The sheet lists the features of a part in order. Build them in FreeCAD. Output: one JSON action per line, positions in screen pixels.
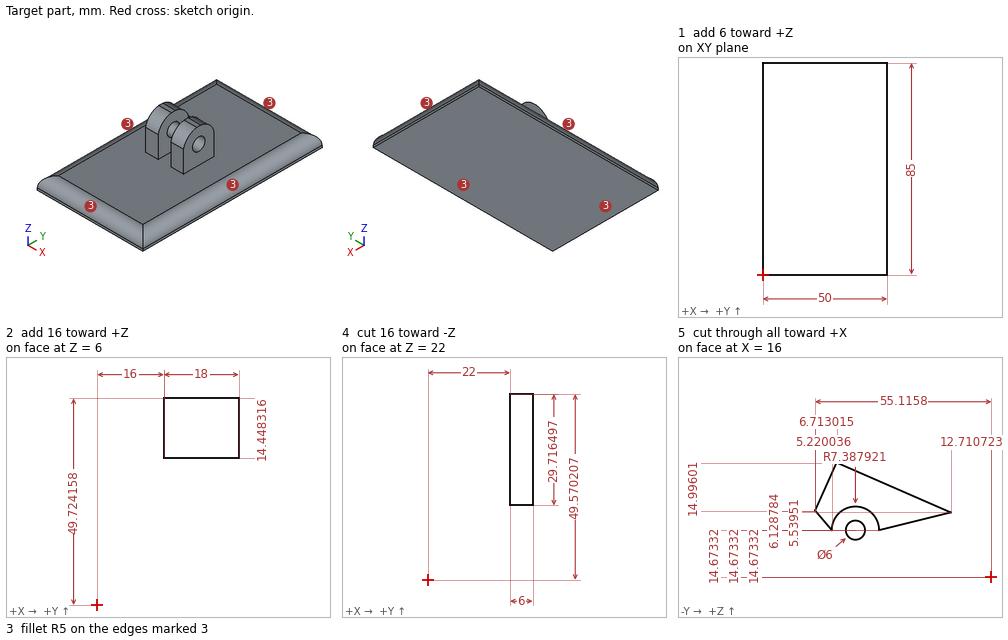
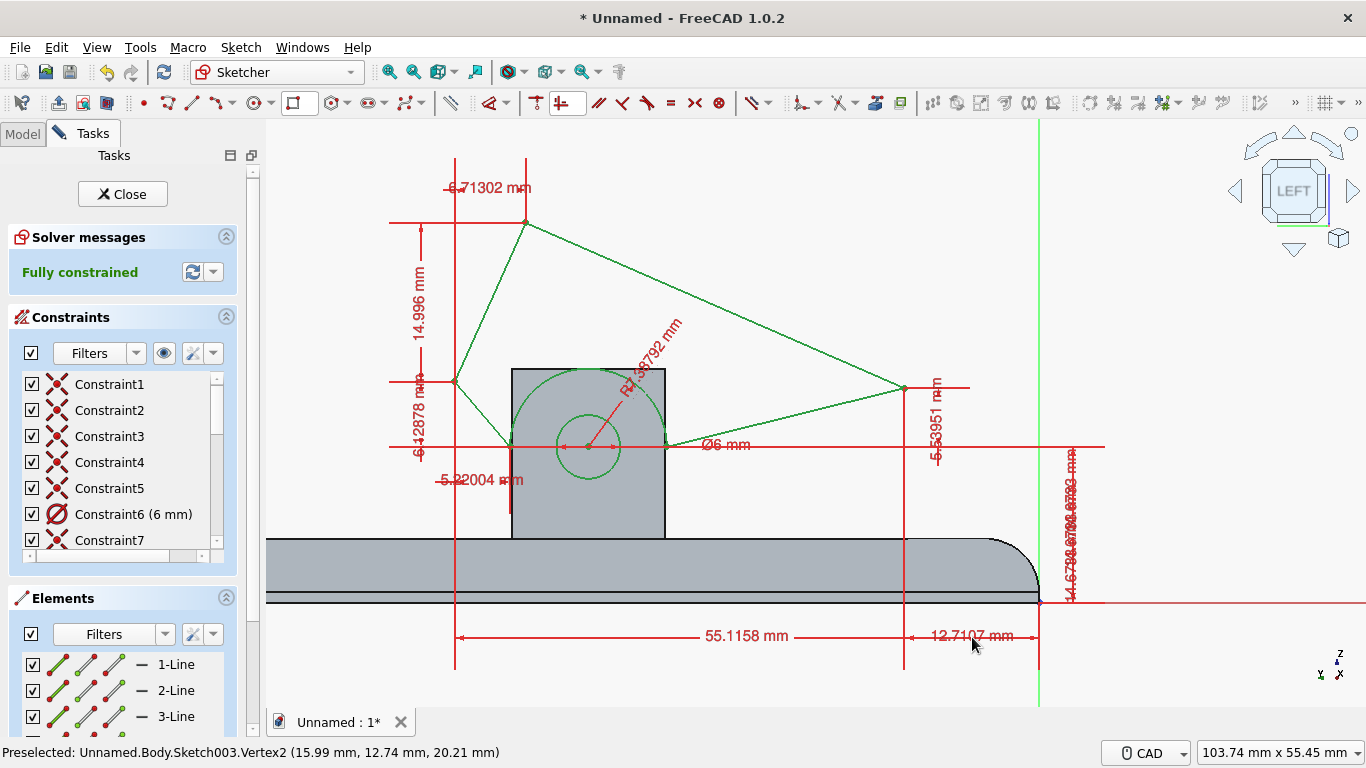
{"action": "left_click", "coordinate": [123, 194]}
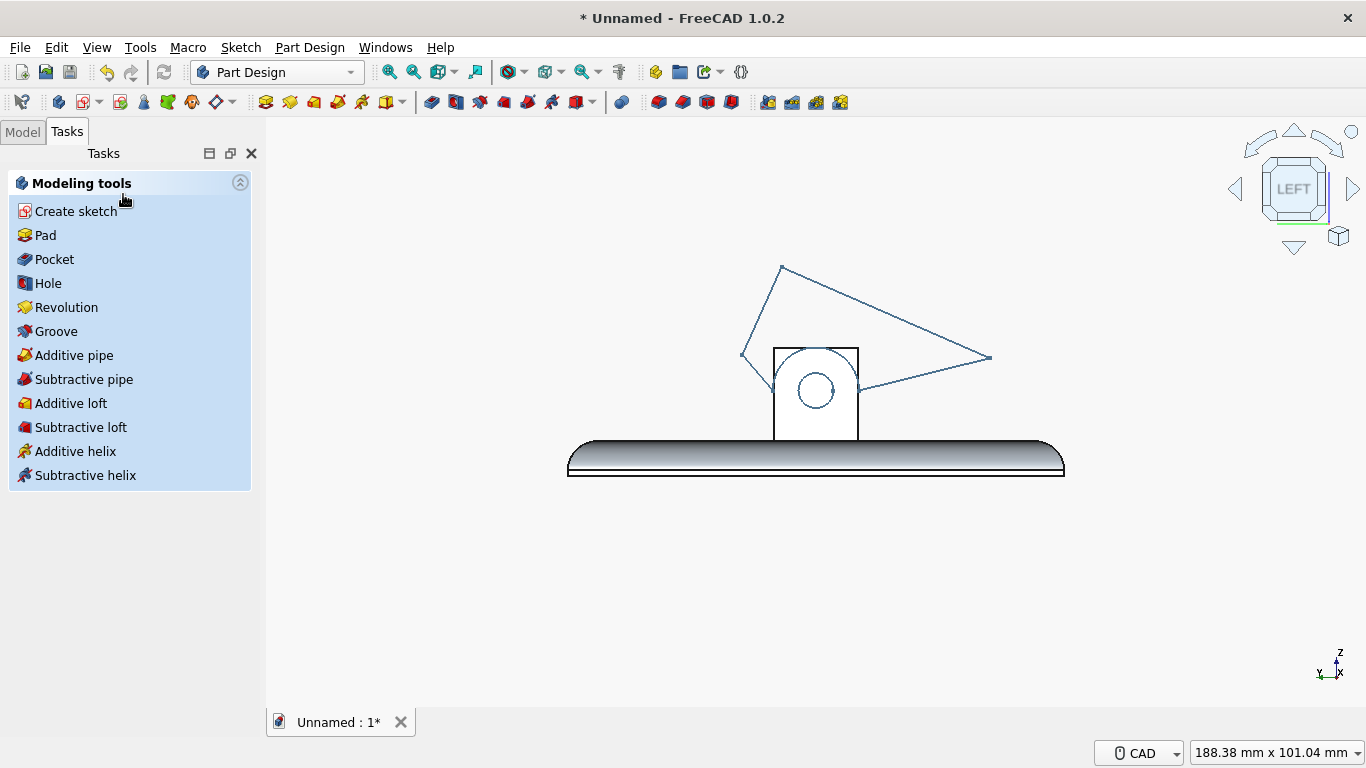
{"action": "left_click", "coordinate": [432, 102]}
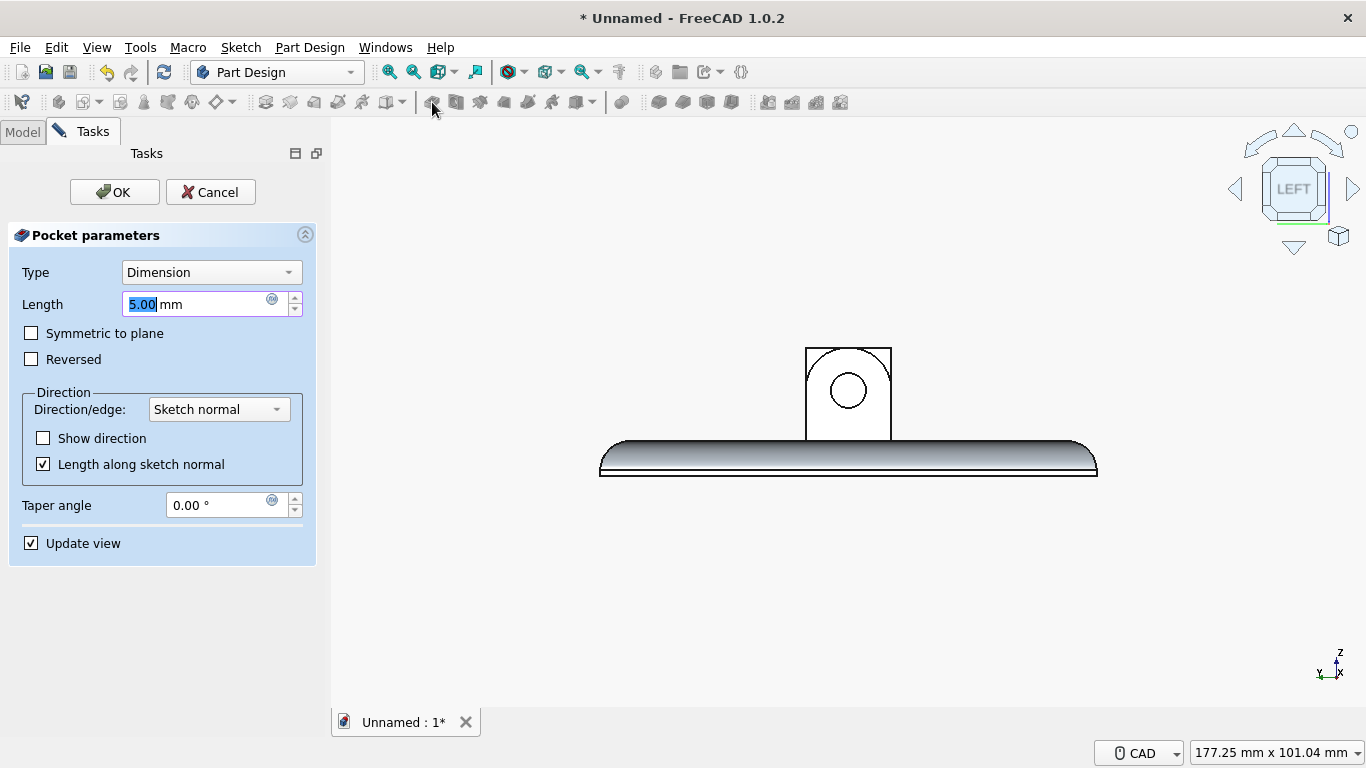
{"action": "left_click", "coordinate": [212, 272]}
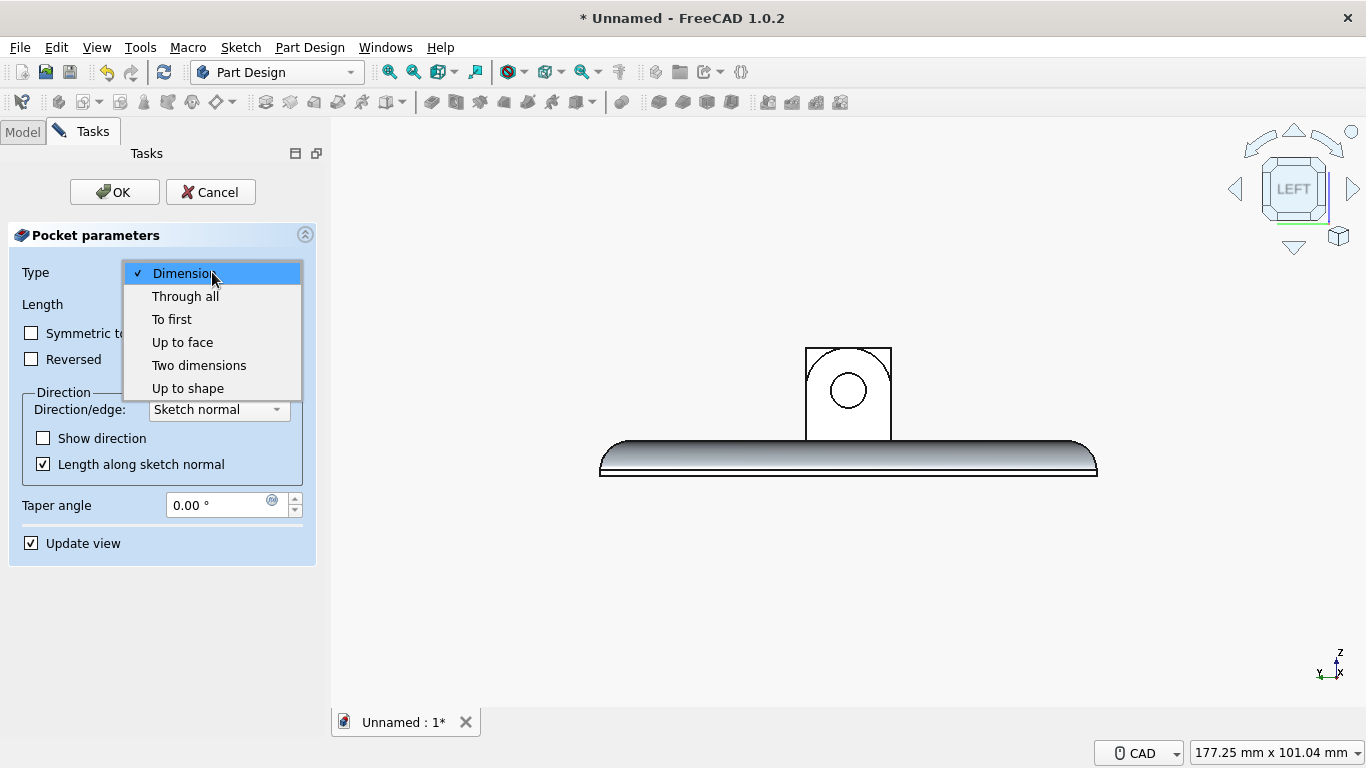
{"action": "left_click", "coordinate": [212, 296]}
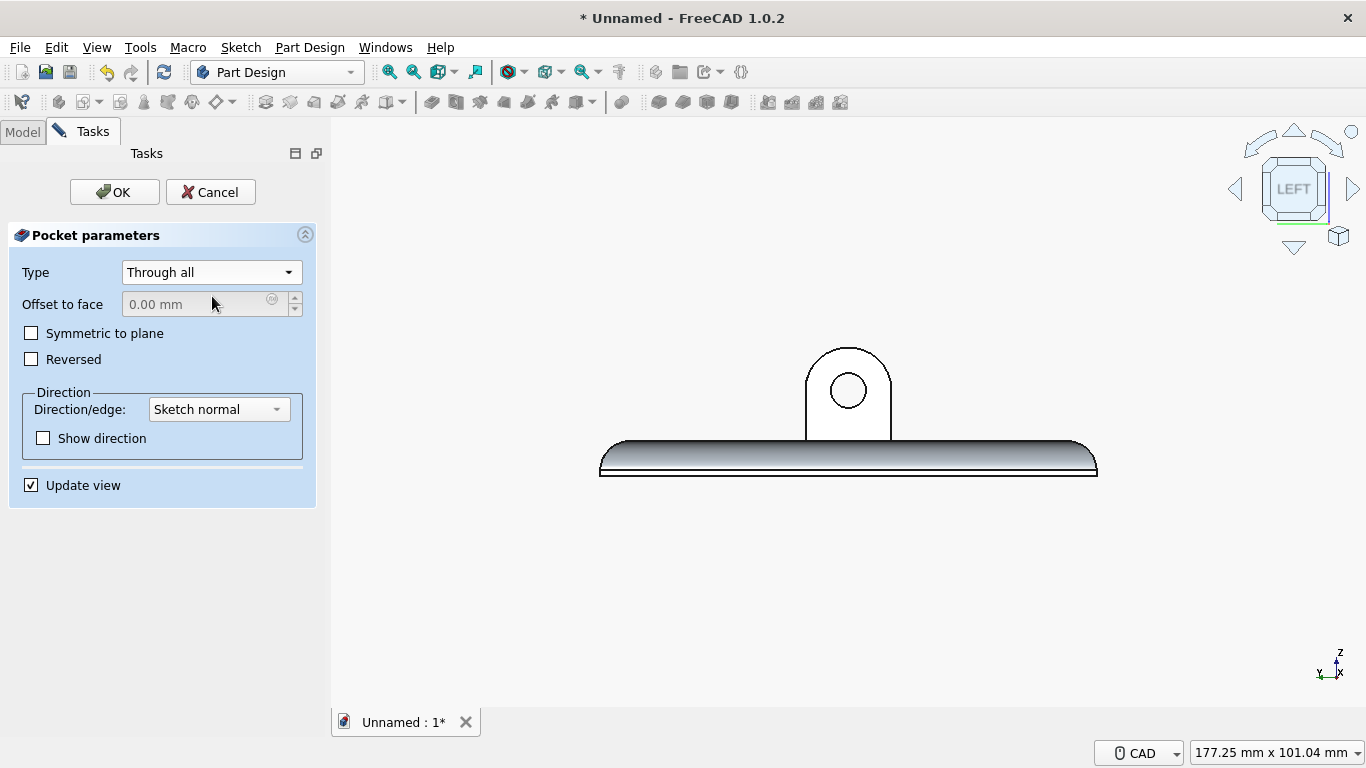
{"action": "left_click", "coordinate": [115, 192]}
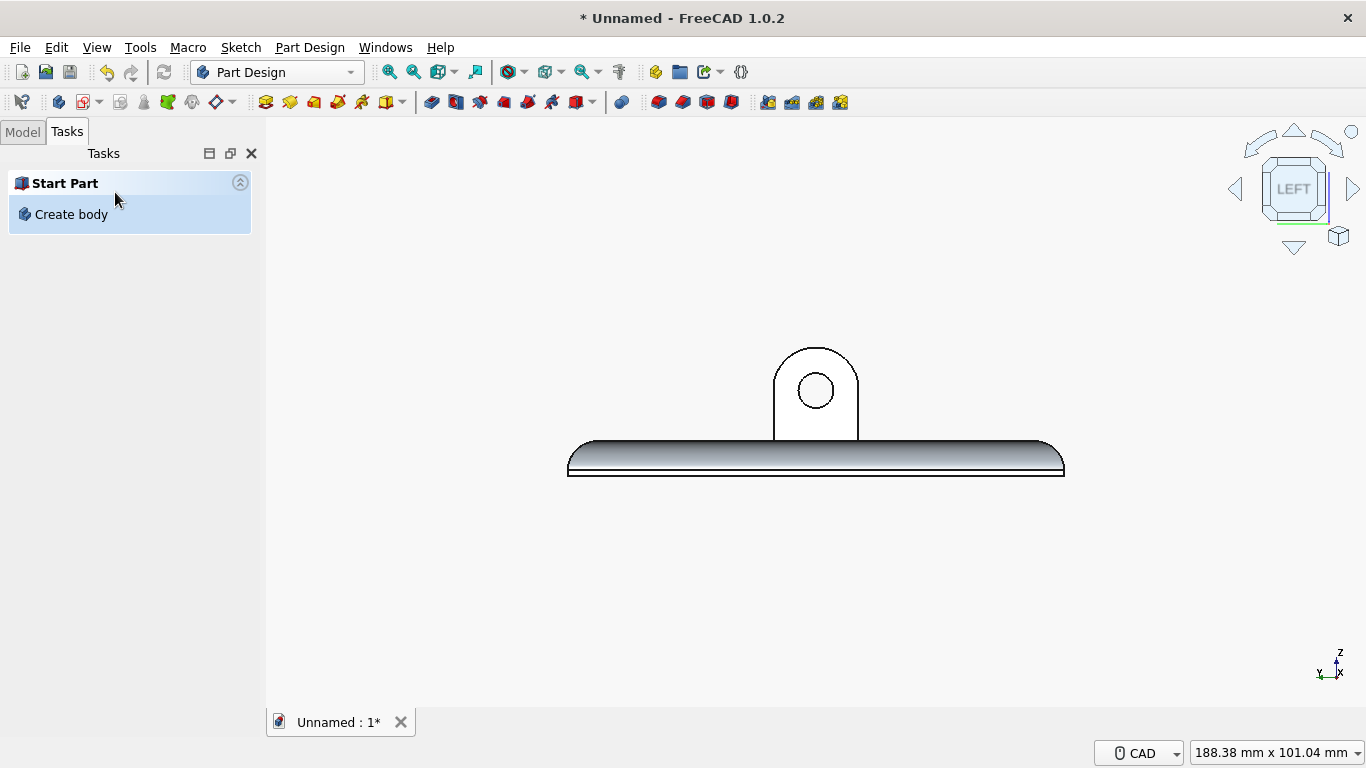
{"action": "key", "text": "0"}